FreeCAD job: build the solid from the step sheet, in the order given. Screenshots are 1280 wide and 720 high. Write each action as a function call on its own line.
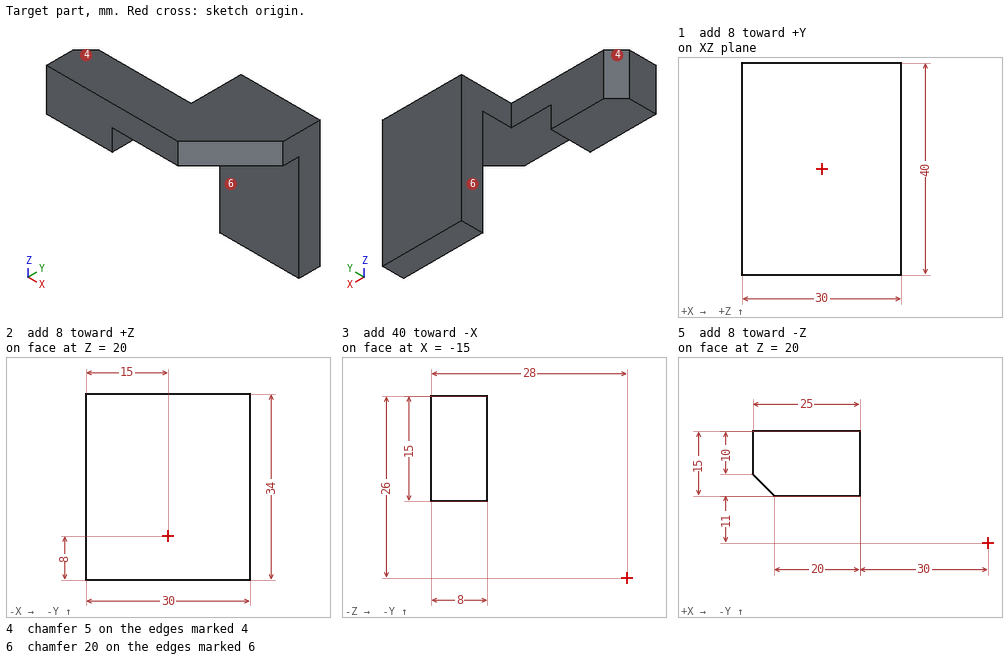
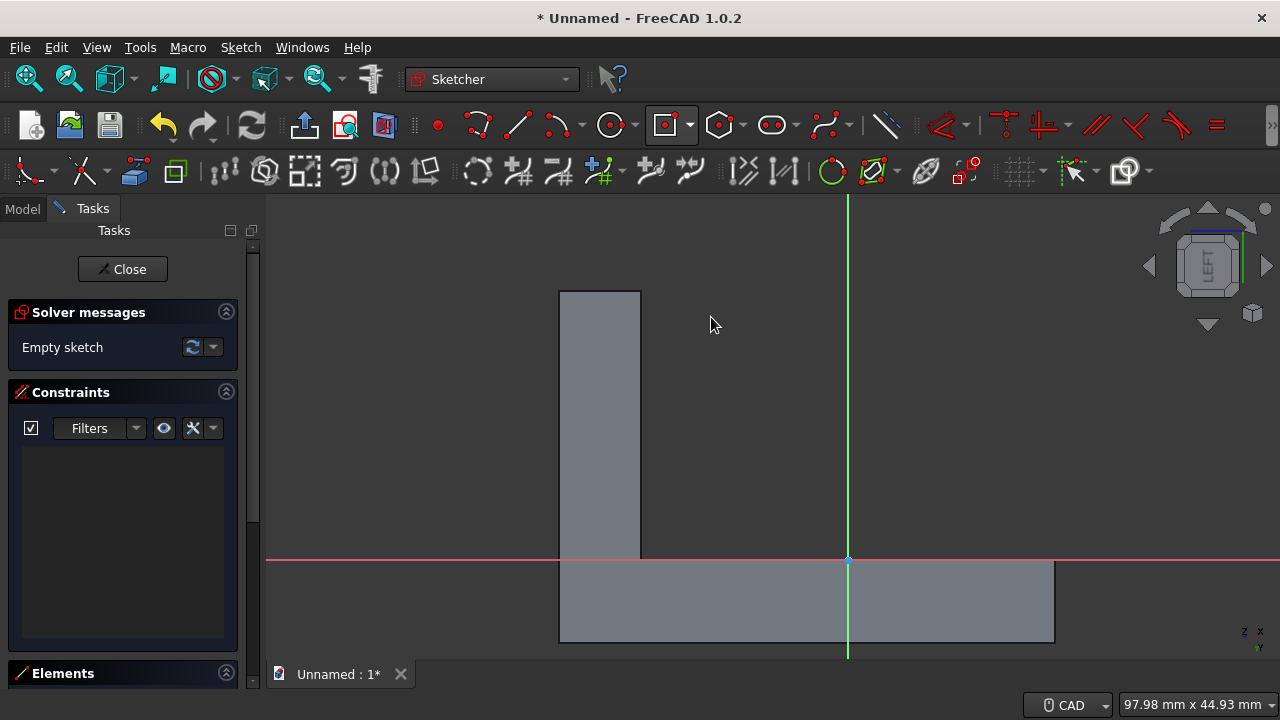
key(g)
key(r)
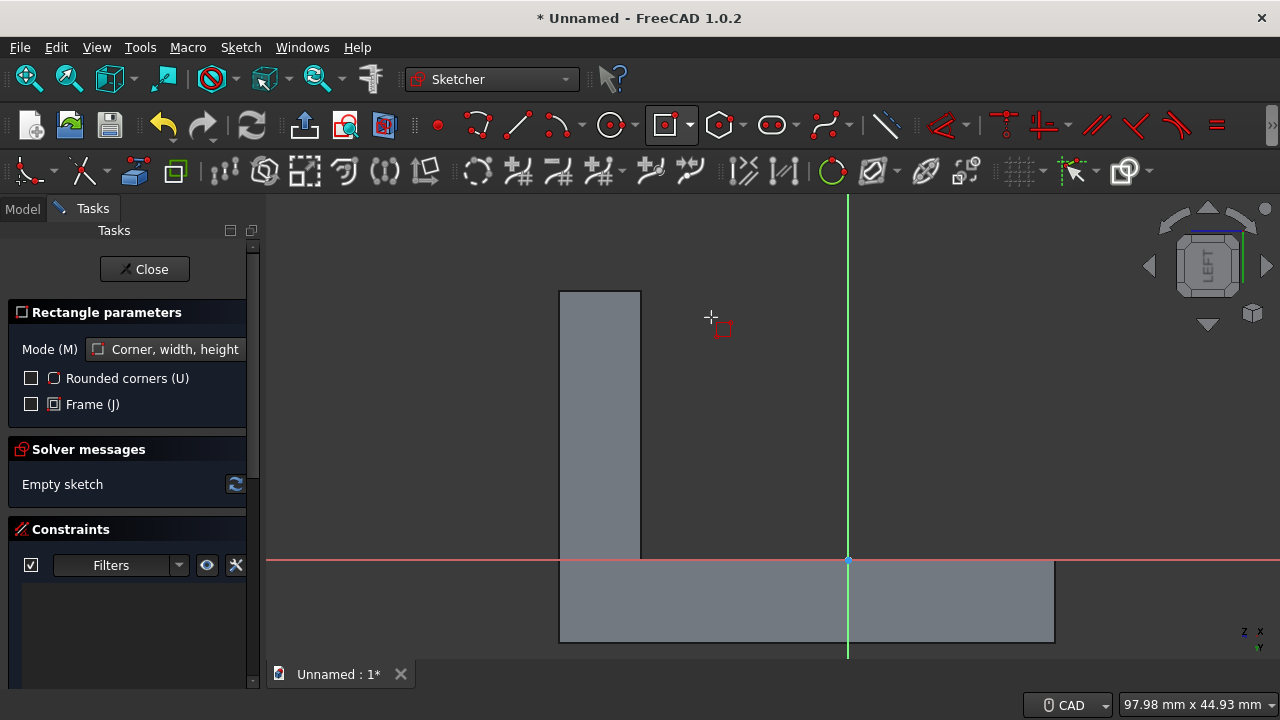
click(559, 291)
move(641, 447)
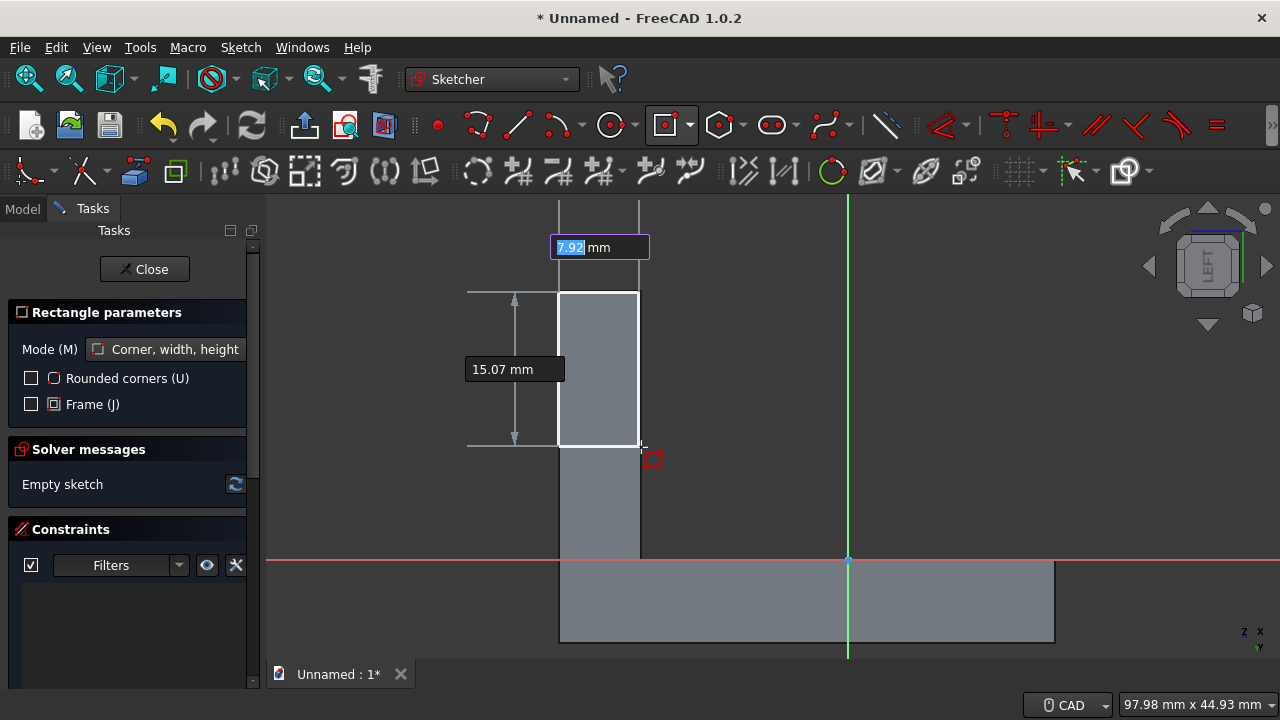
text(8)
key(Tab)
text(15)
key(Return)
key(Escape)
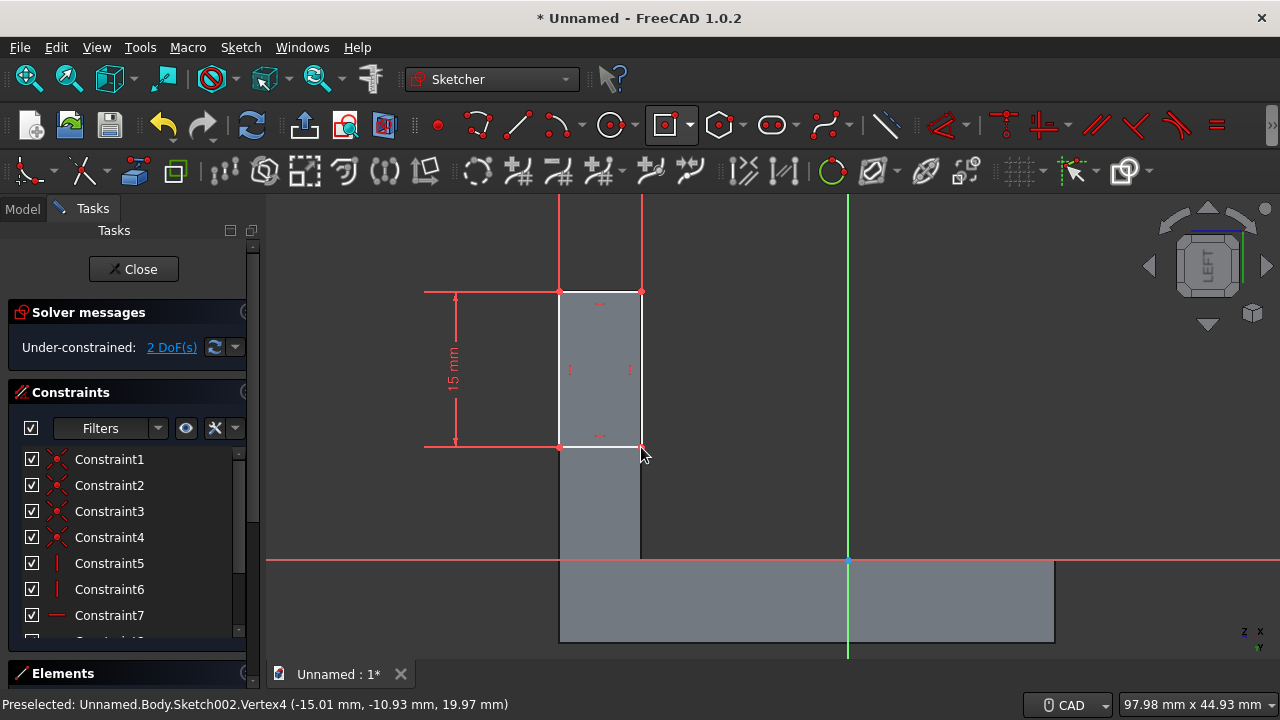
click(942, 126)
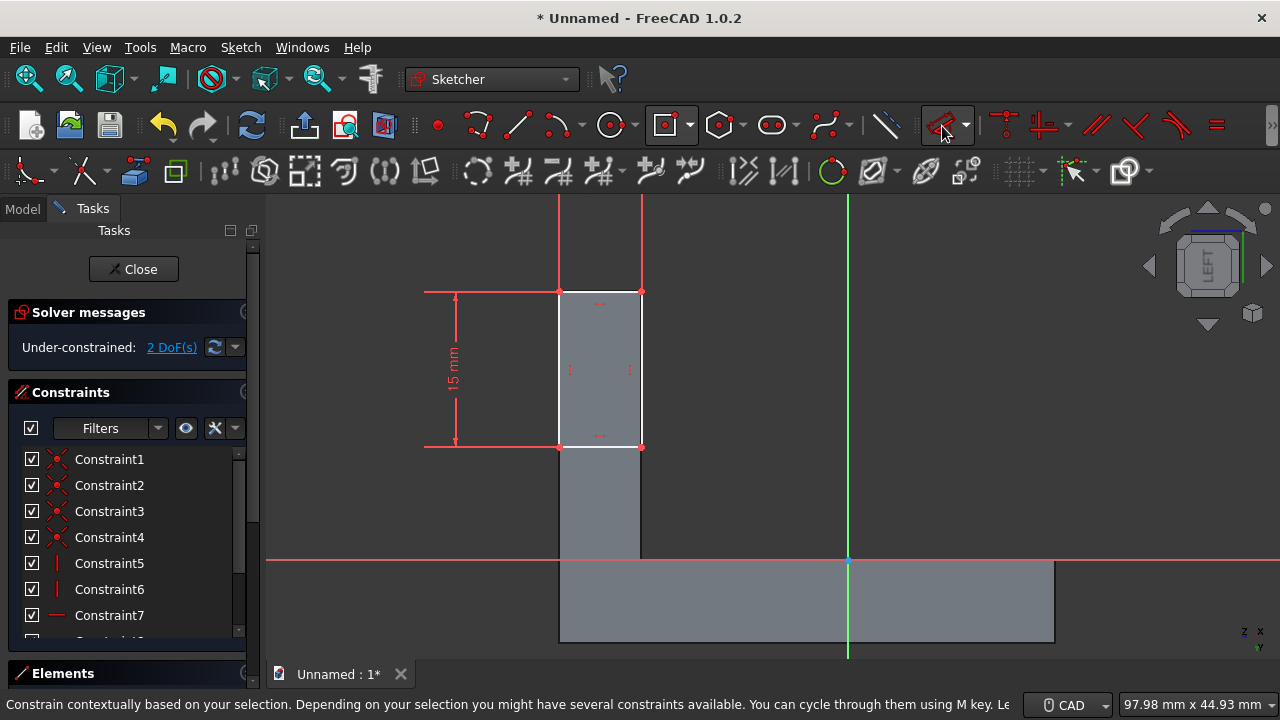
click(559, 292)
click(704, 594)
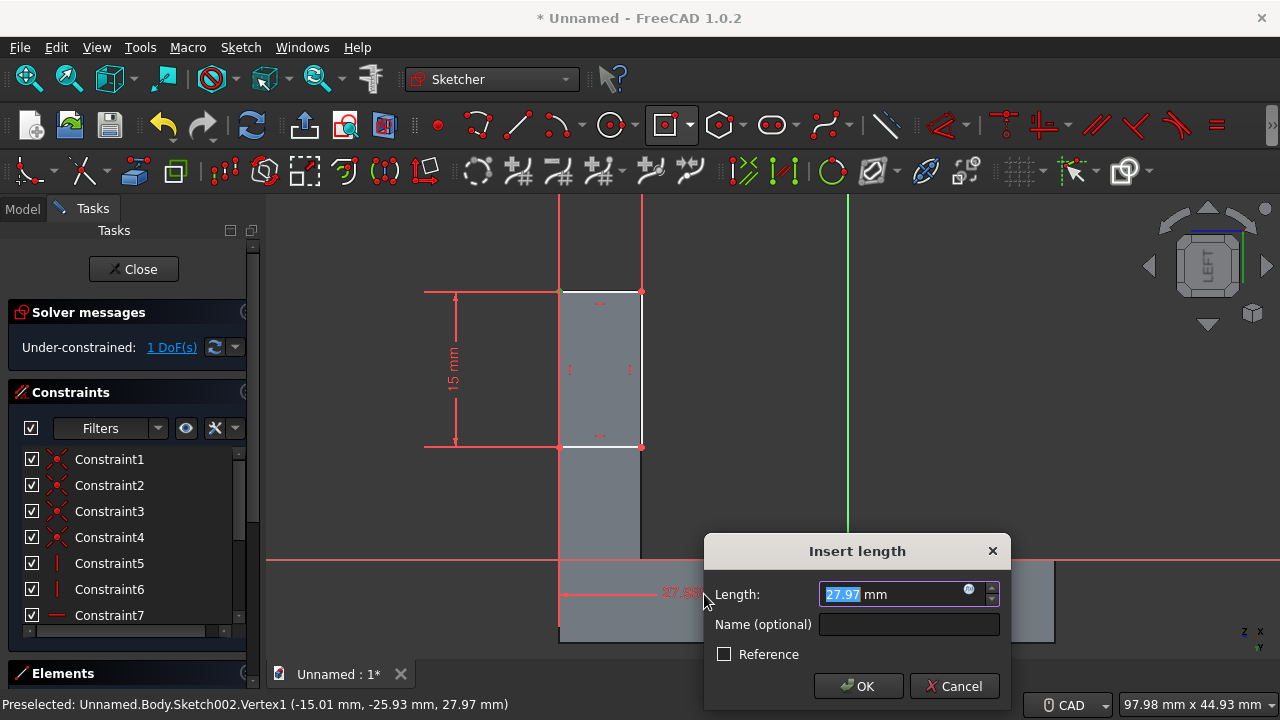
text(28)
key(Return)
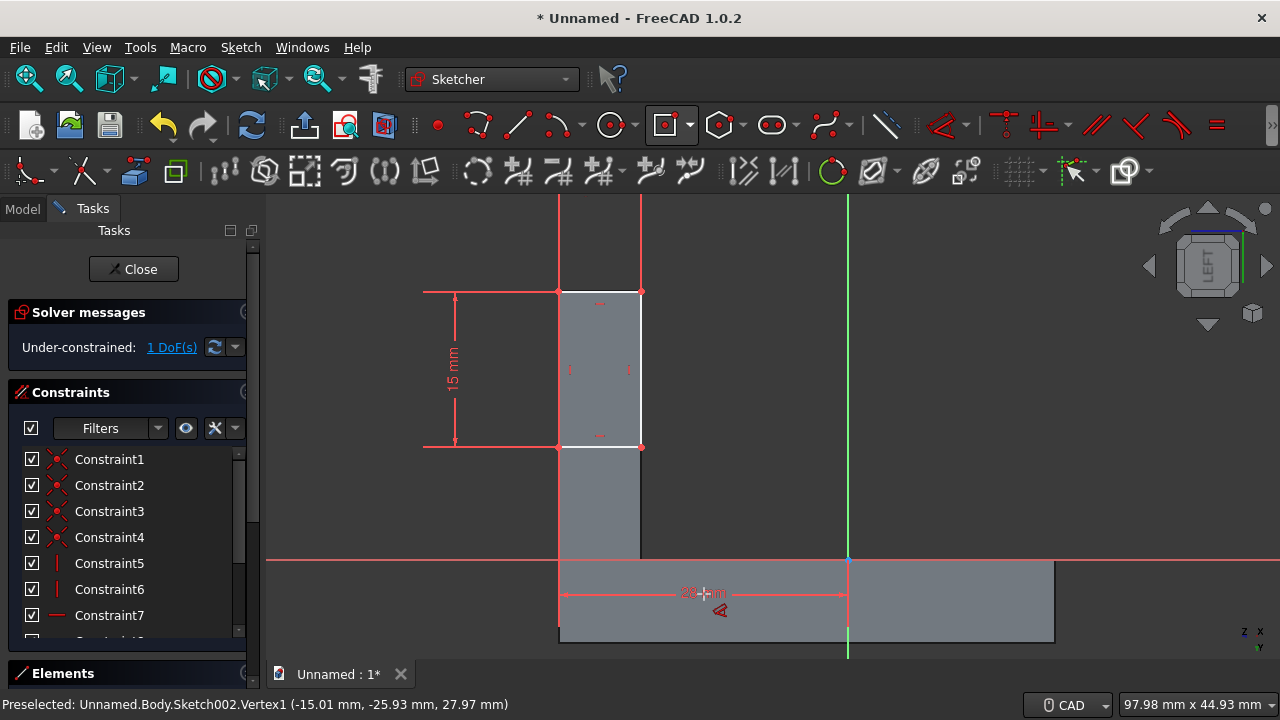
click(559, 292)
click(882, 426)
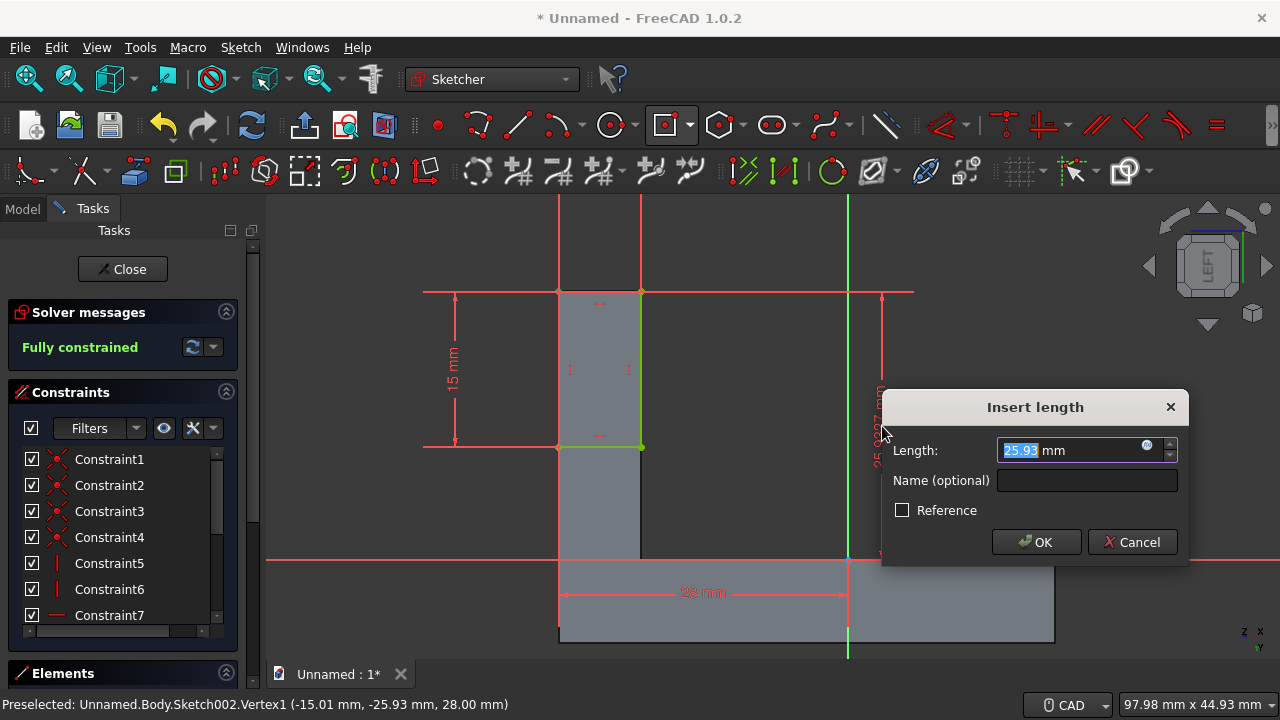
text(26)
key(Return)
key(Escape)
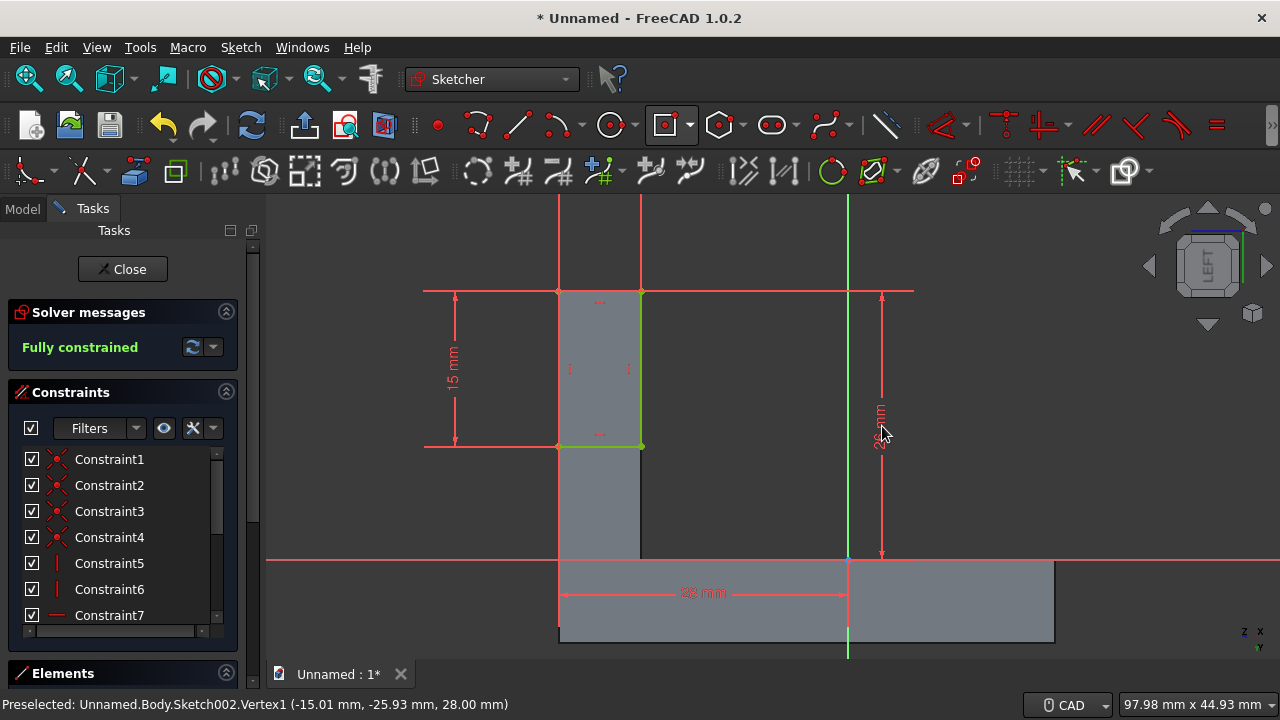
click(123, 269)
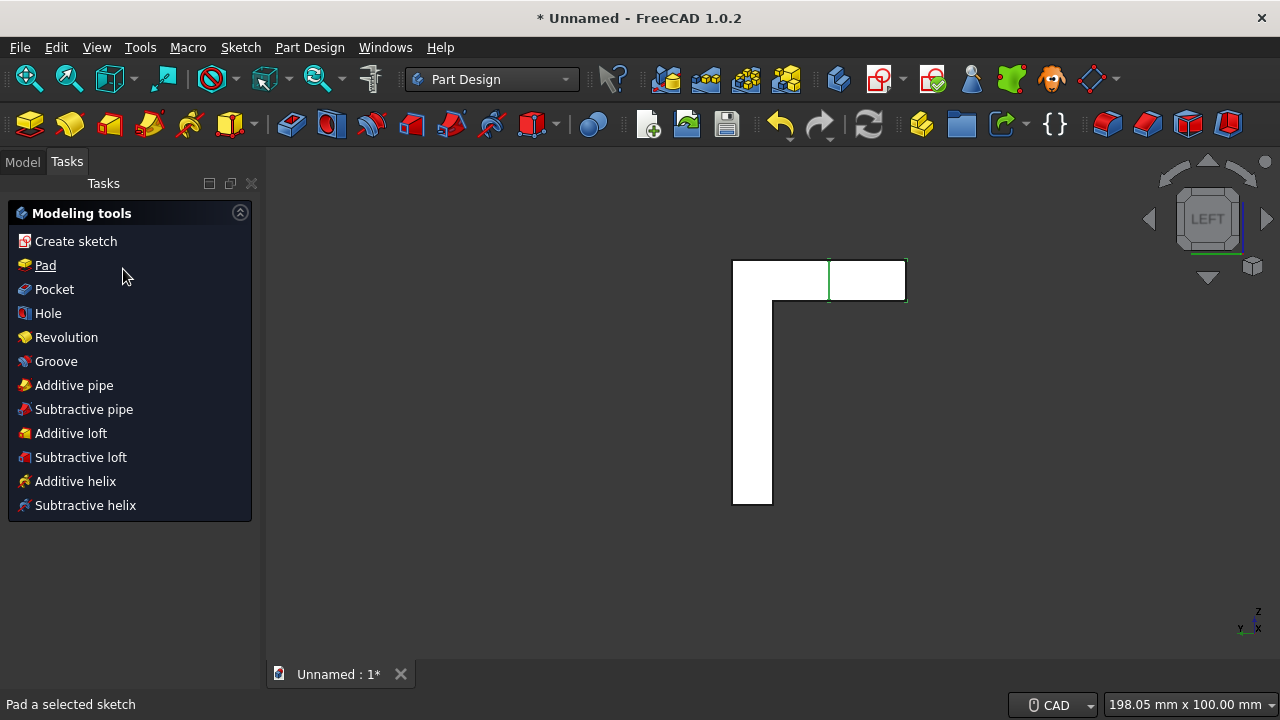
click(30, 124)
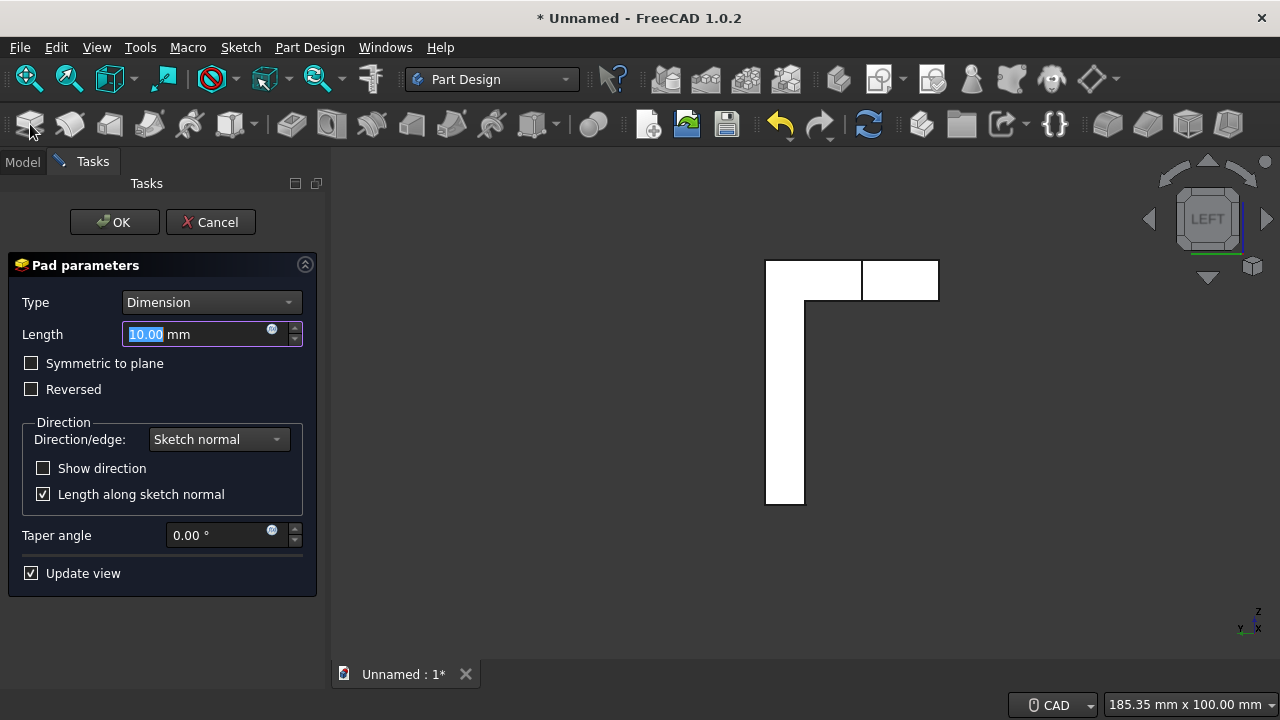
text(40)
key(Tab)